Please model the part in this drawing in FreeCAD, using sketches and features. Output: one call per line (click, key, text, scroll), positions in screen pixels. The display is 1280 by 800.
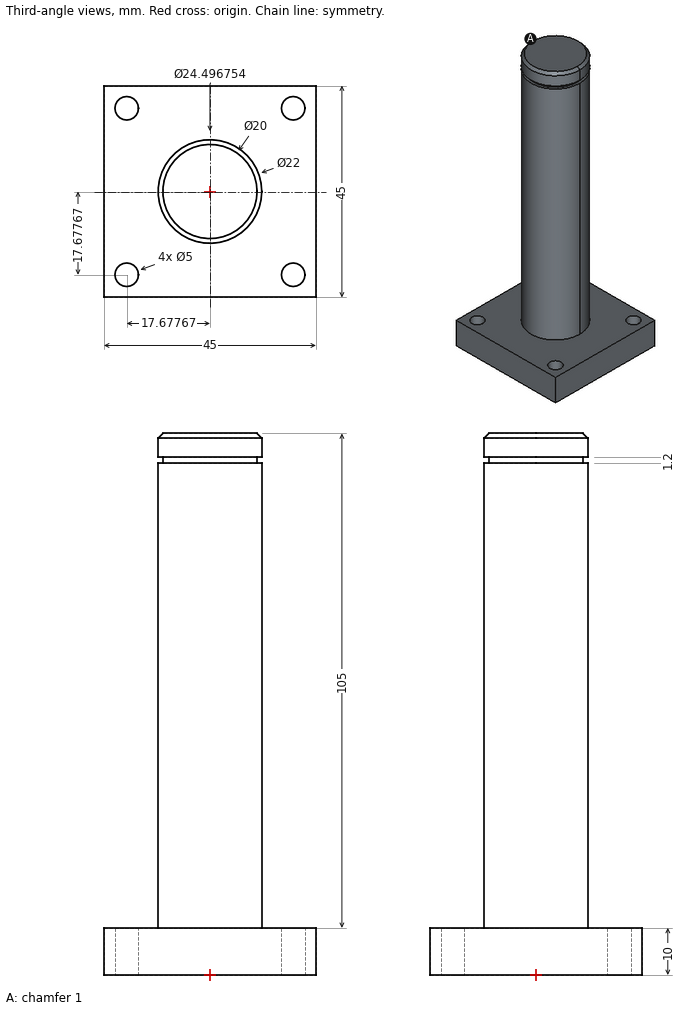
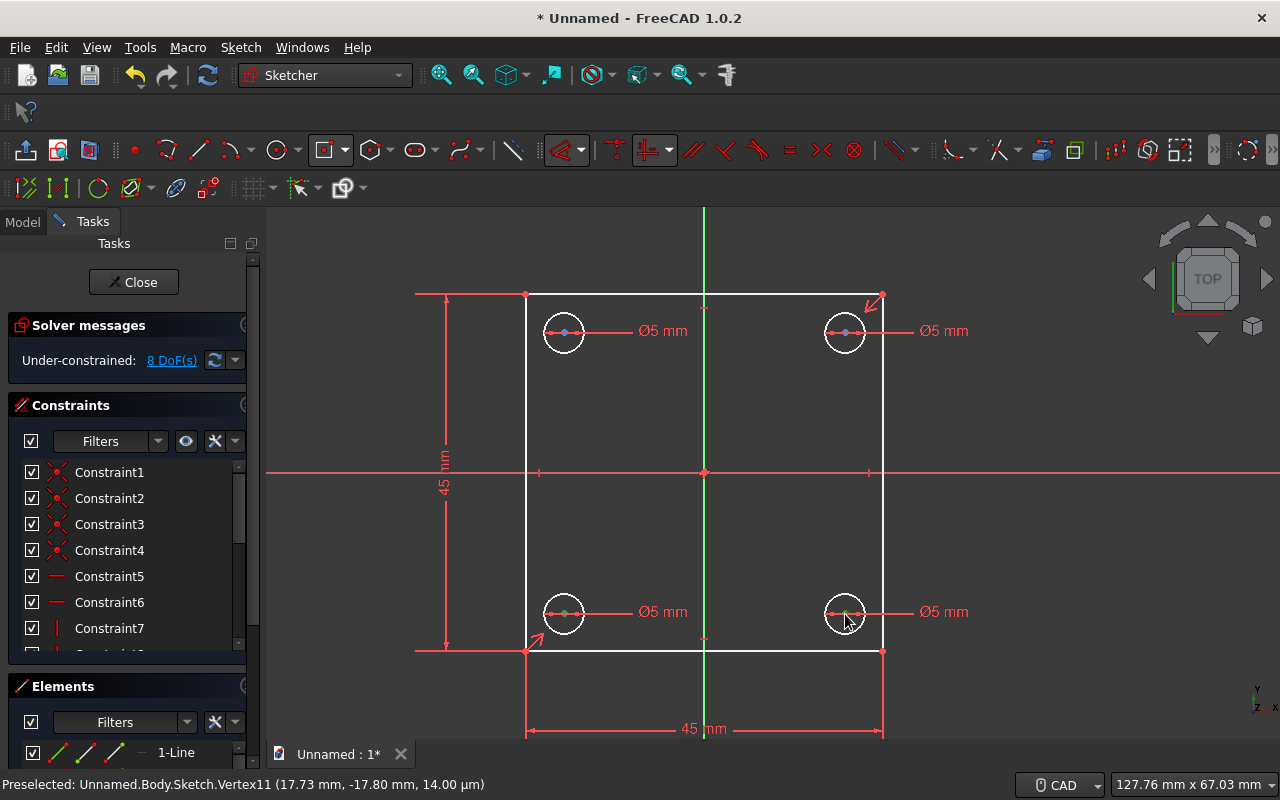
click(704, 609)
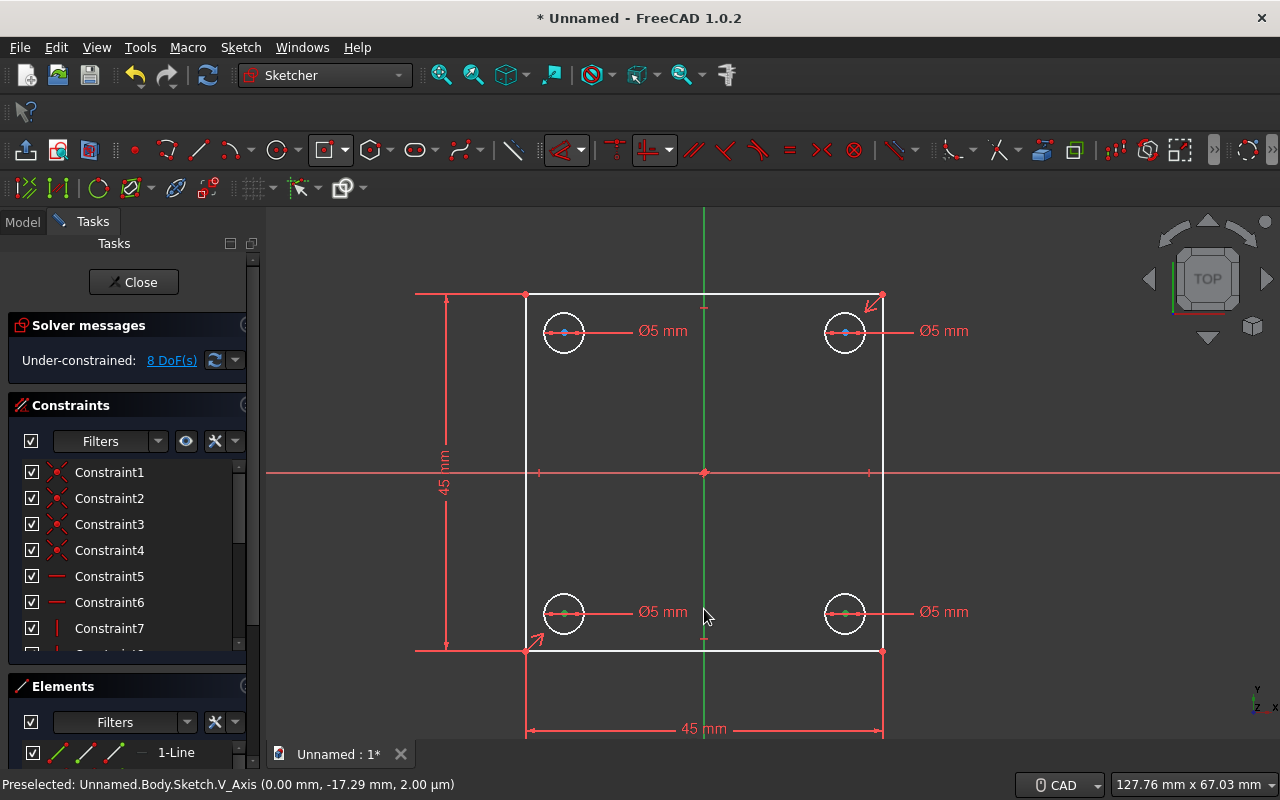
click(822, 150)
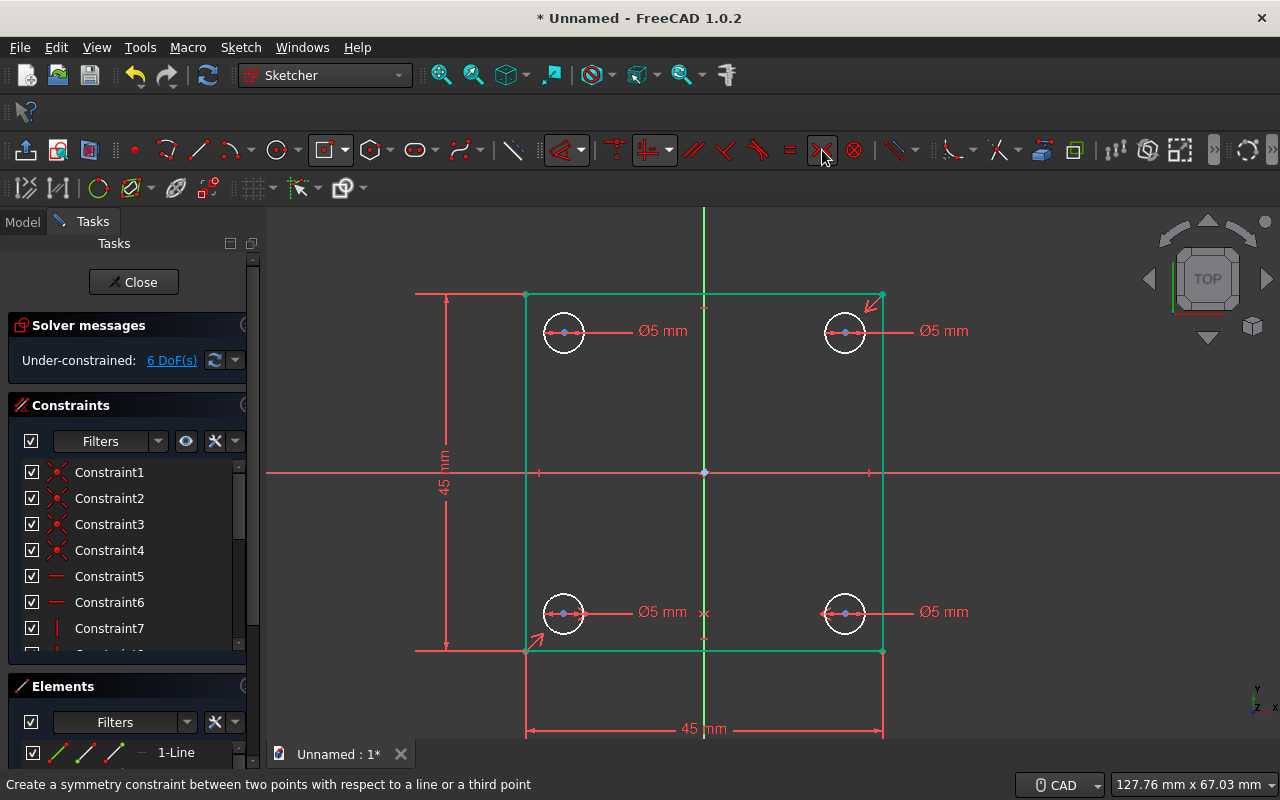
click(564, 614)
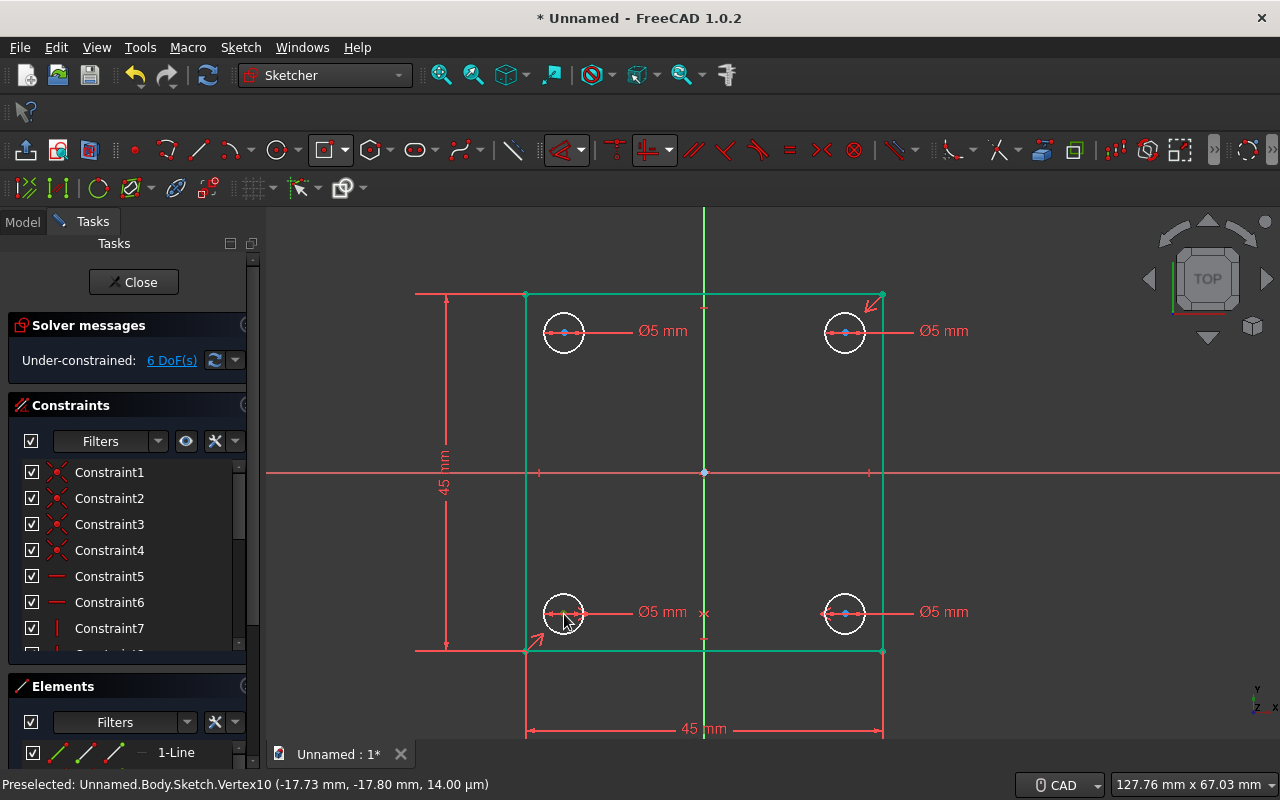
click(564, 333)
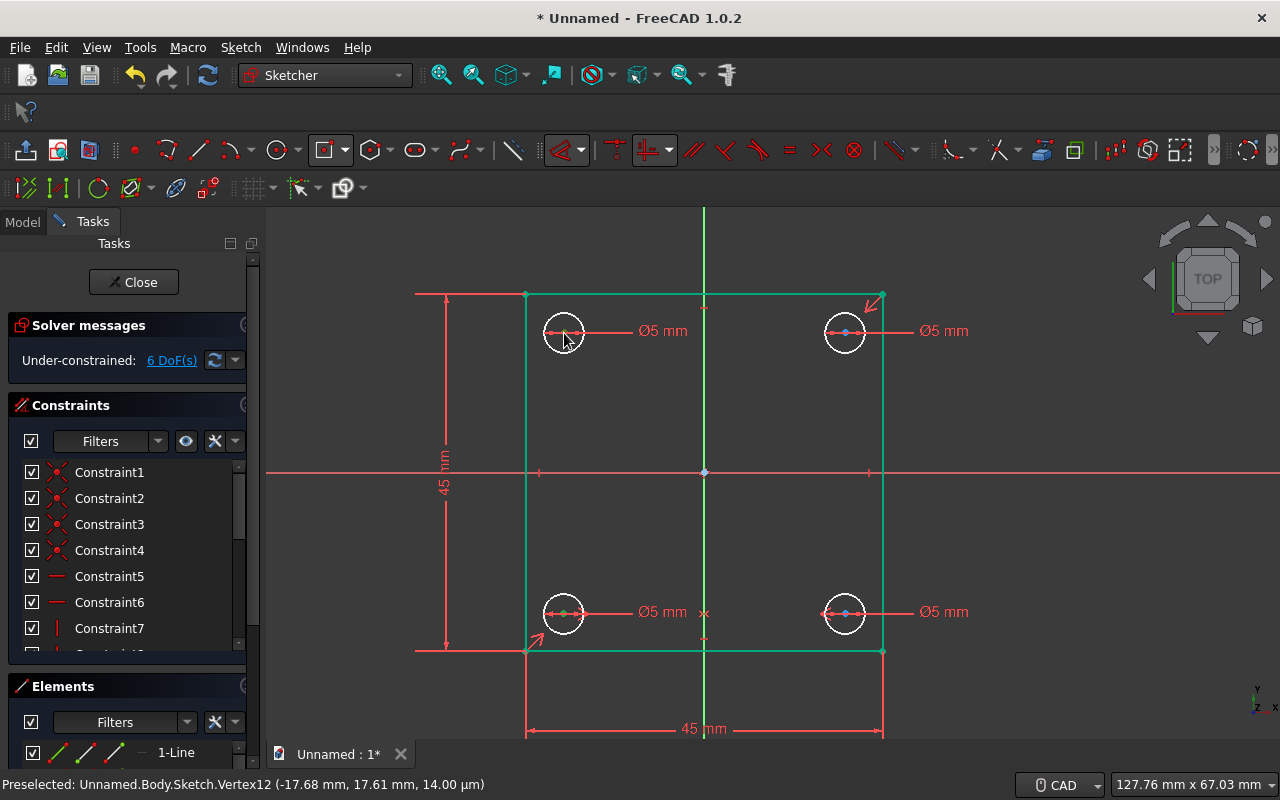
click(353, 473)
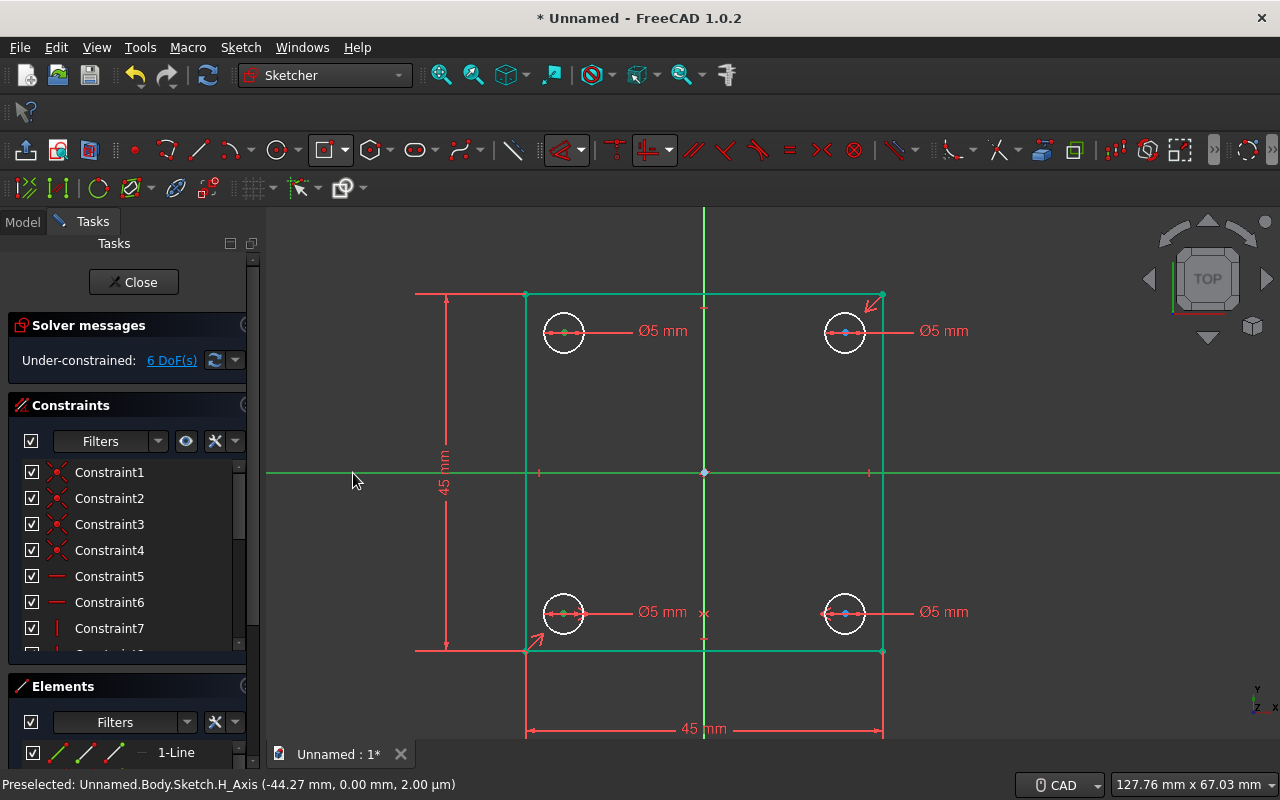
click(822, 150)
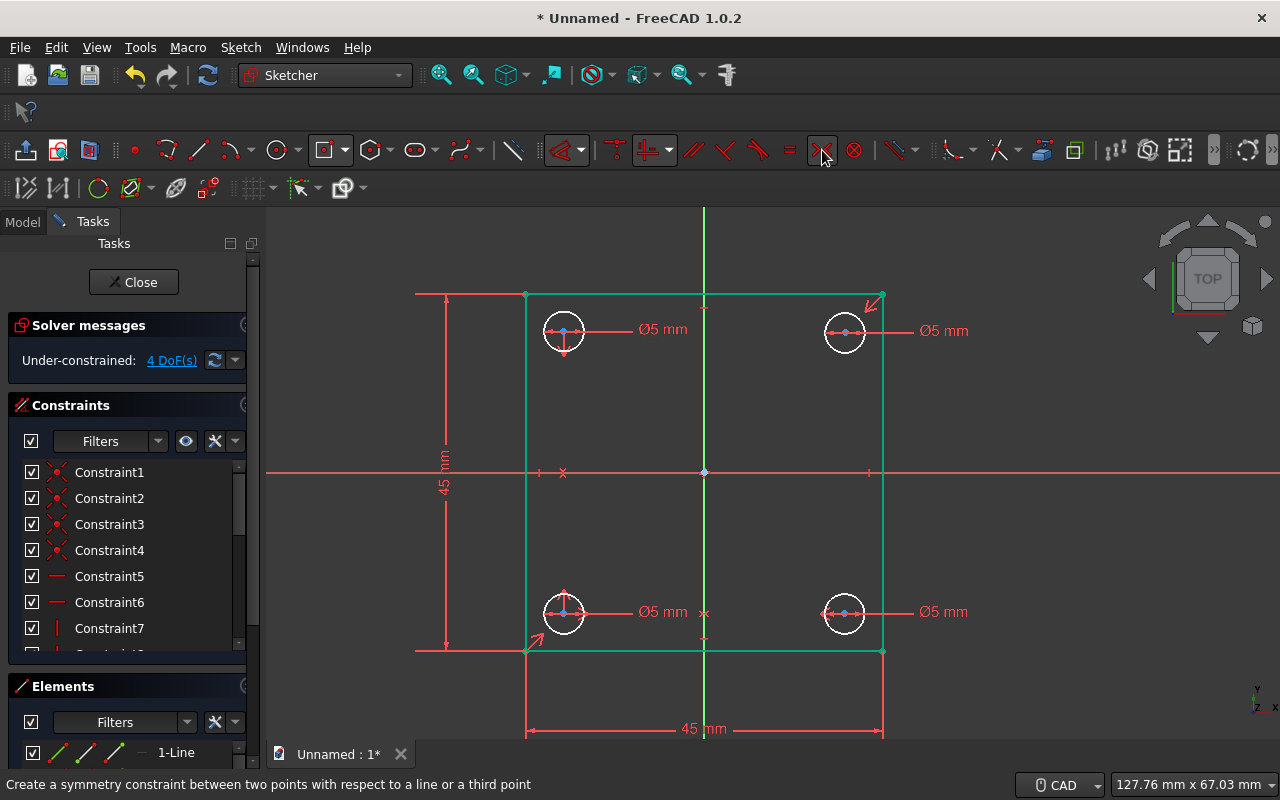
click(845, 614)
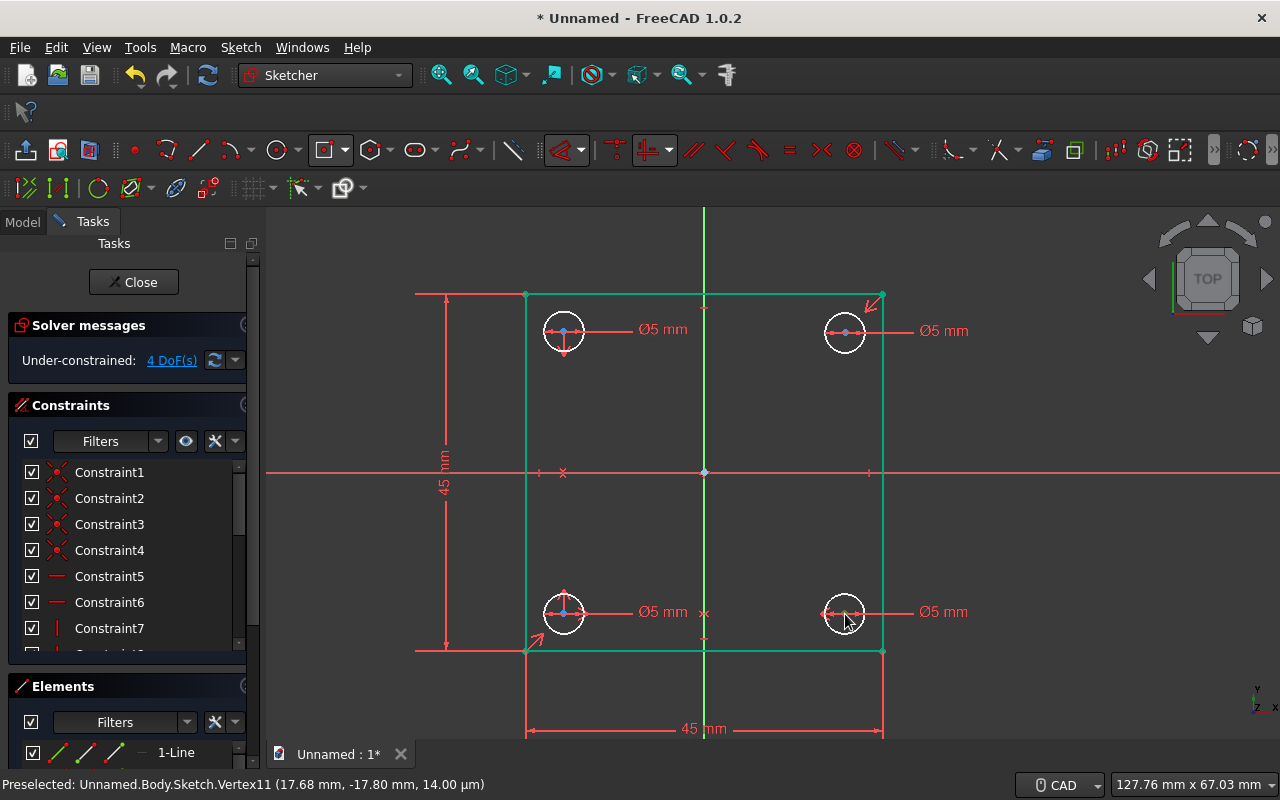
click(845, 333)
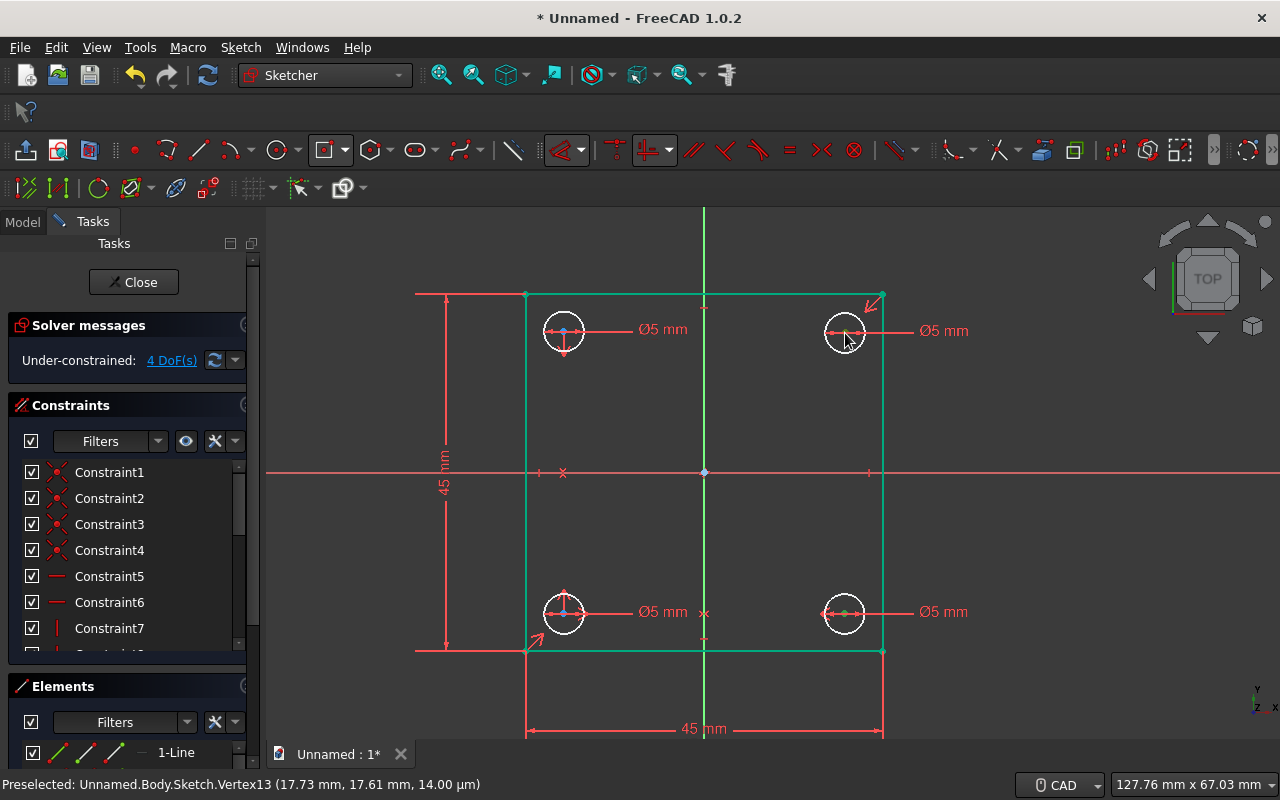
click(353, 473)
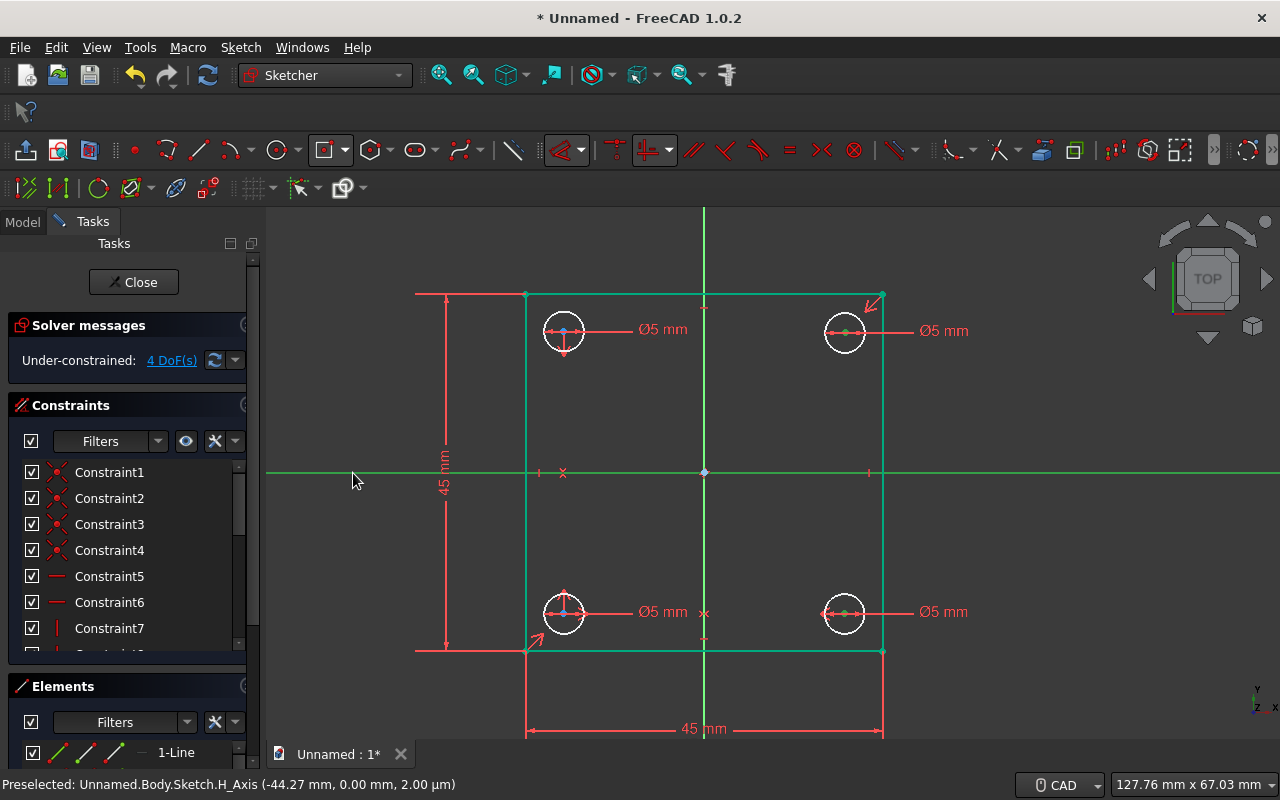
click(822, 150)